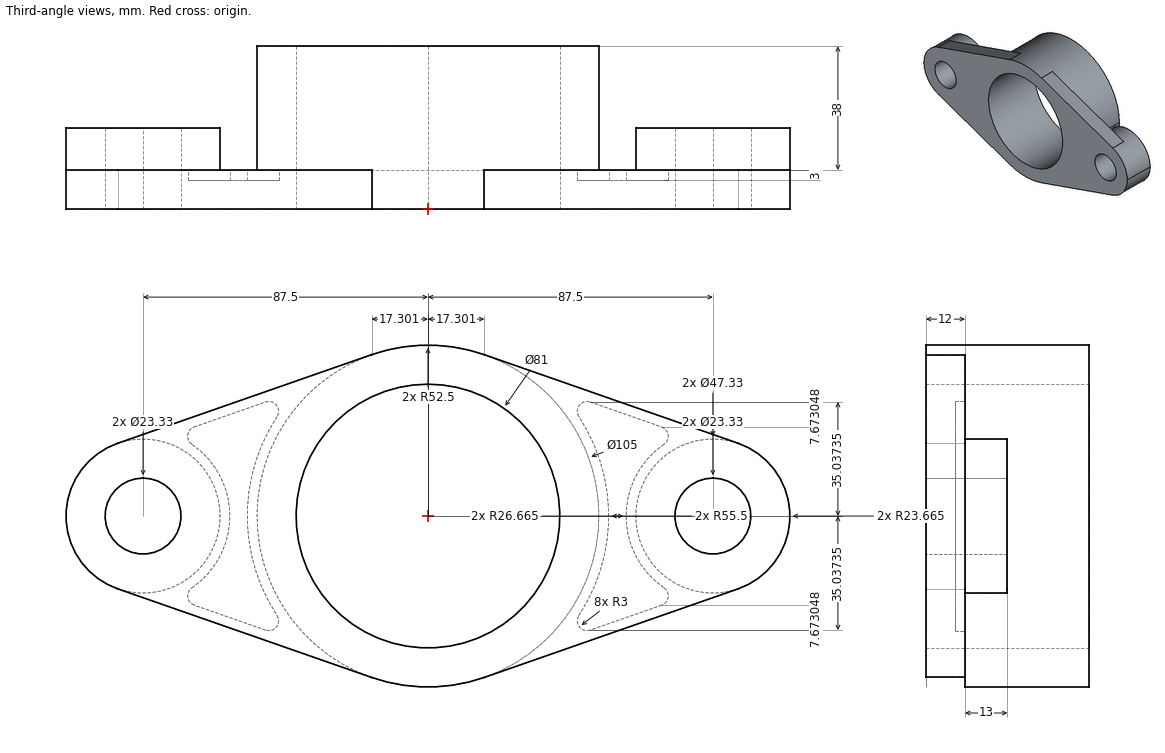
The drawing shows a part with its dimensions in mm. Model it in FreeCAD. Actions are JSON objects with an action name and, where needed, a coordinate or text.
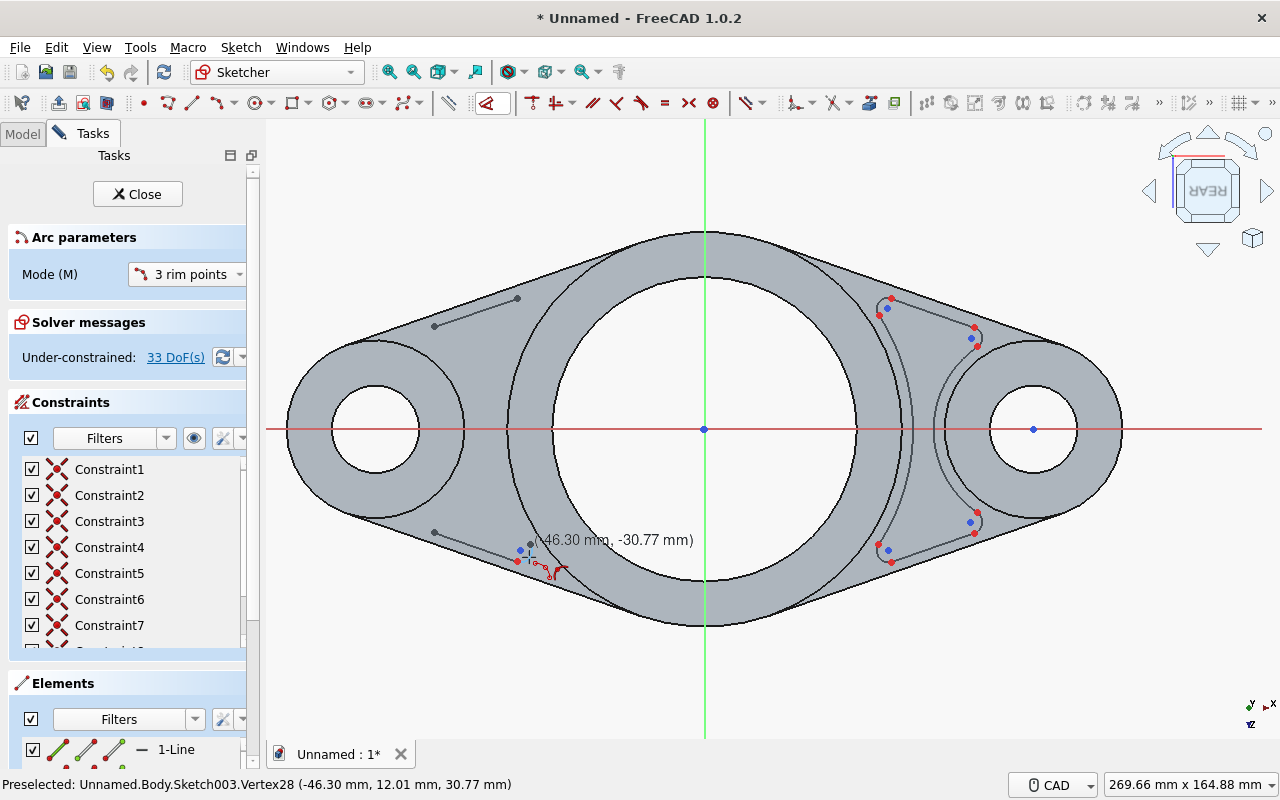
{"action": "left_click", "coordinate": [530, 314]}
{"action": "left_click", "coordinate": [497, 405]}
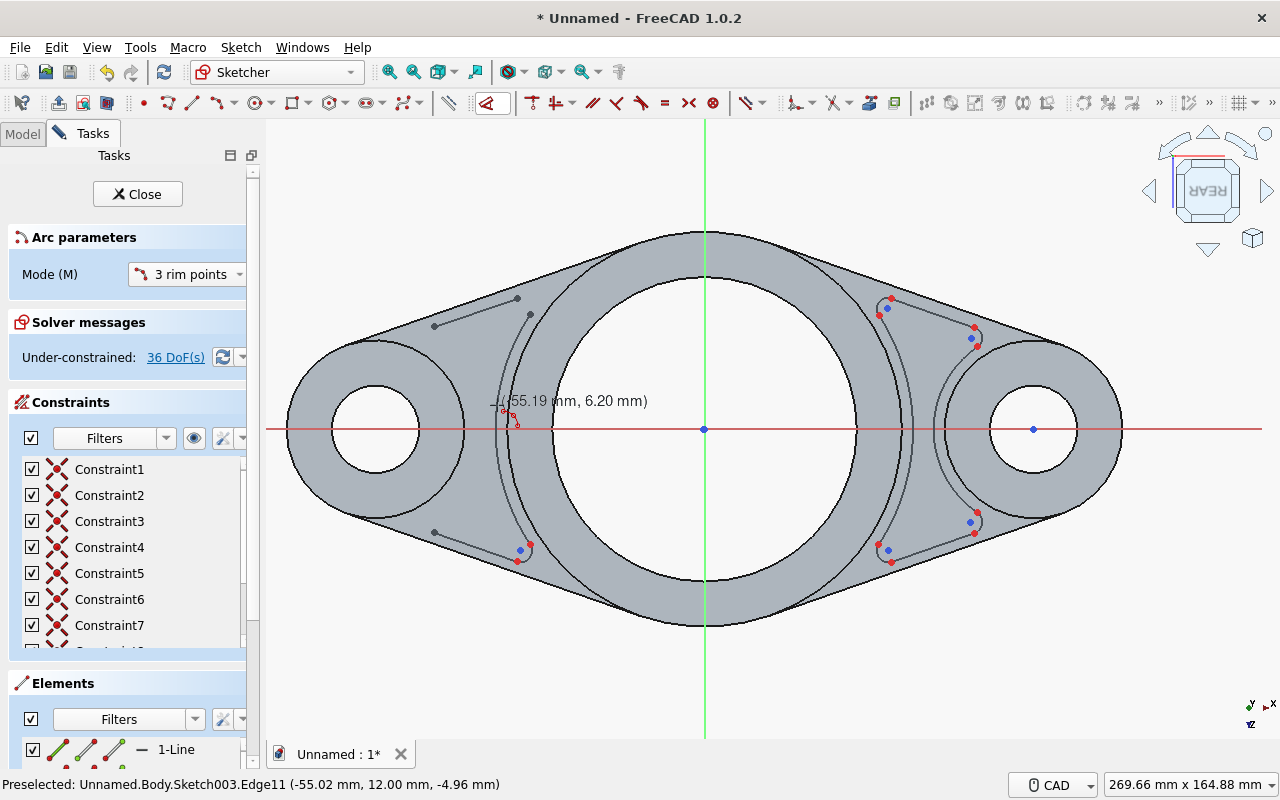
{"action": "left_click", "coordinate": [530, 315]}
{"action": "left_click", "coordinate": [517, 299]}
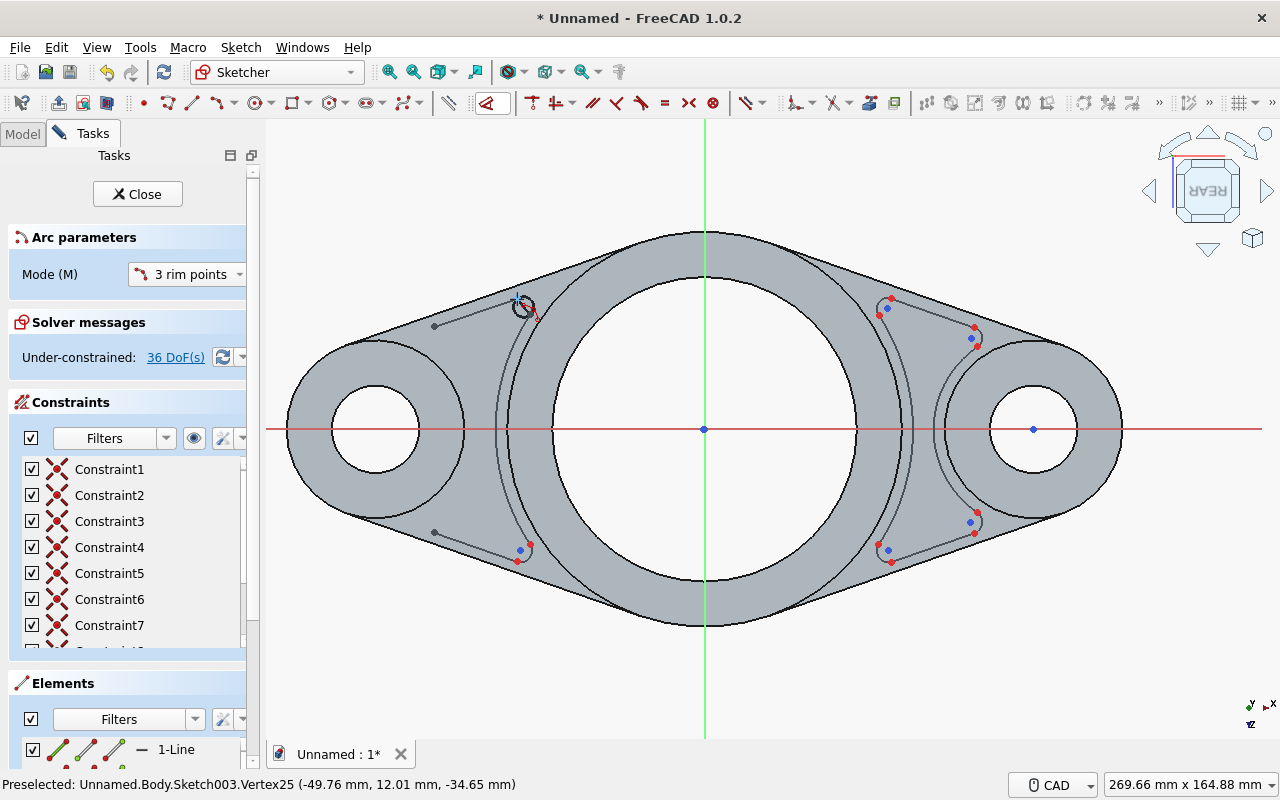
{"action": "scroll", "coordinate": [530, 301], "scroll_direction": "up", "scroll_amount": 4}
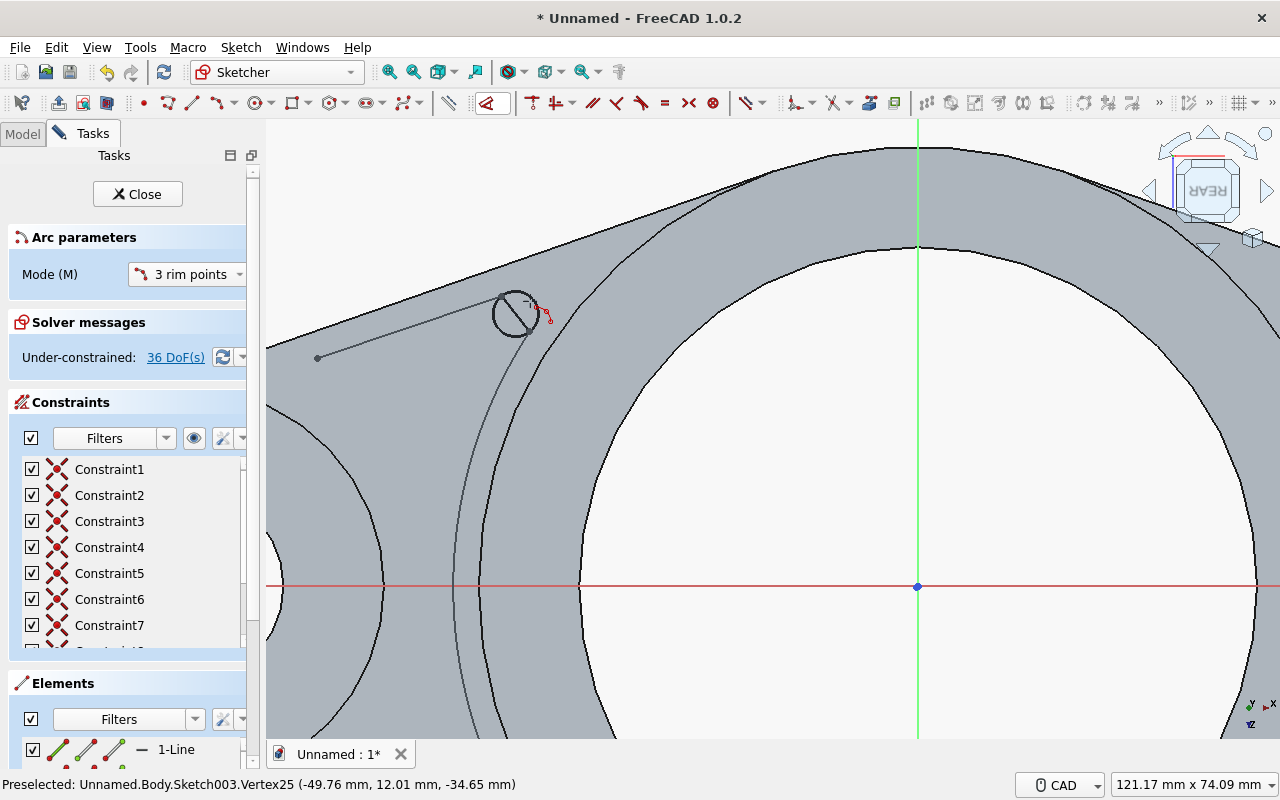
{"action": "left_click", "coordinate": [529, 301]}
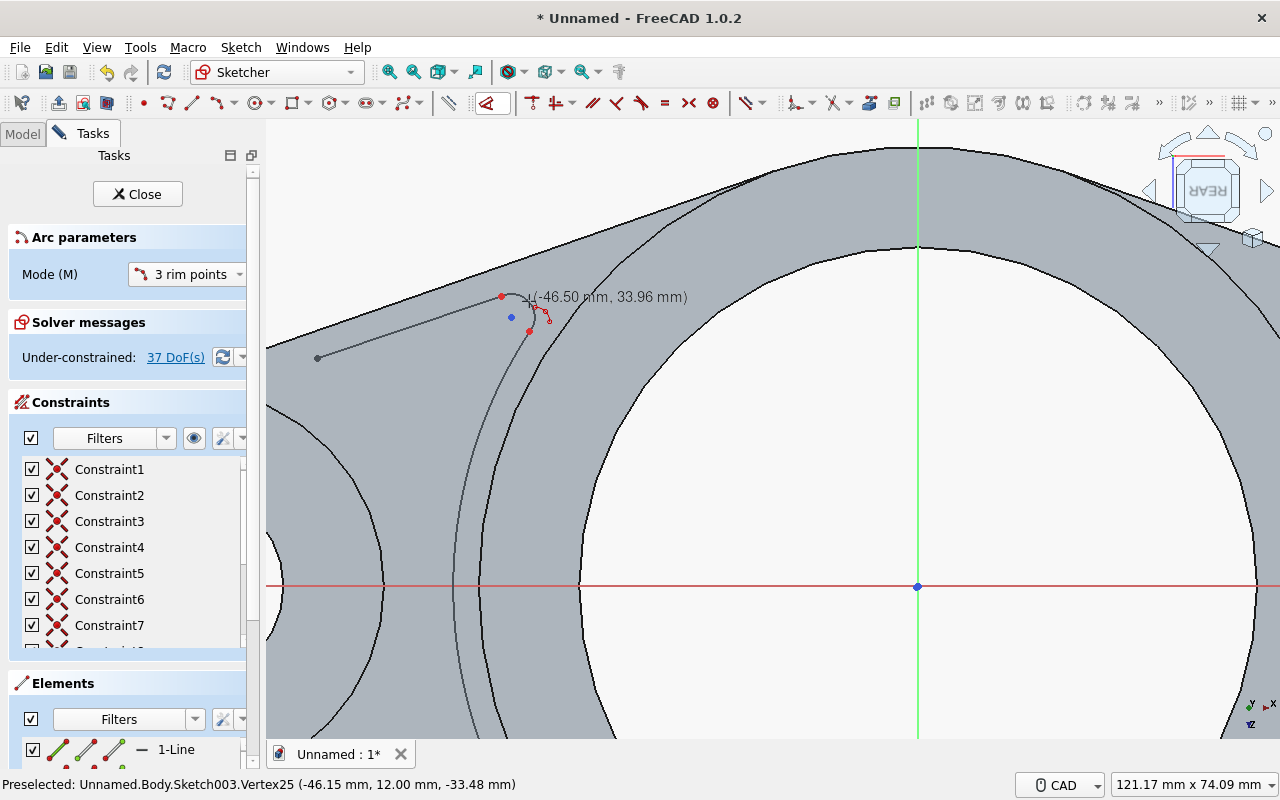
{"action": "left_click", "coordinate": [317, 359]}
{"action": "left_click", "coordinate": [311, 402]}
{"action": "left_click", "coordinate": [301, 378]}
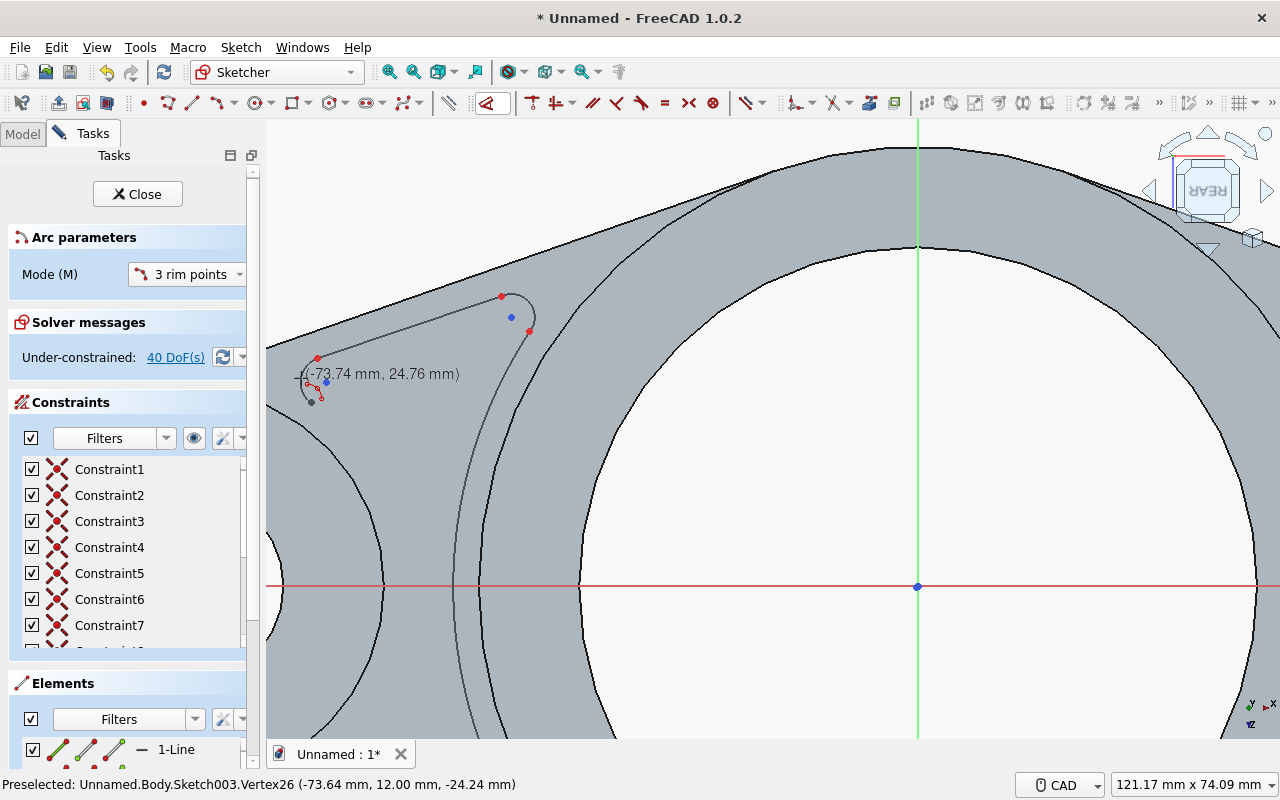
{"action": "left_click", "coordinate": [311, 403]}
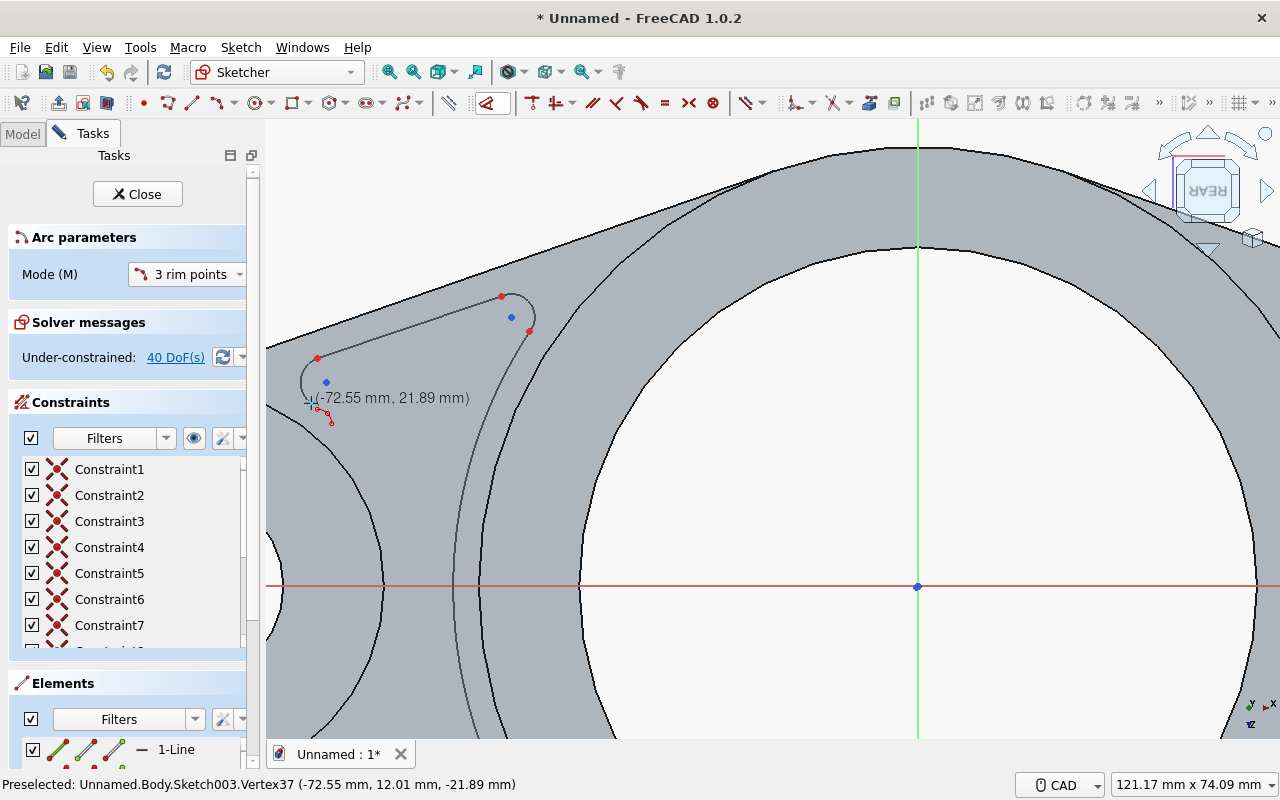
{"action": "scroll", "coordinate": [530, 301], "scroll_direction": "down", "scroll_amount": 4}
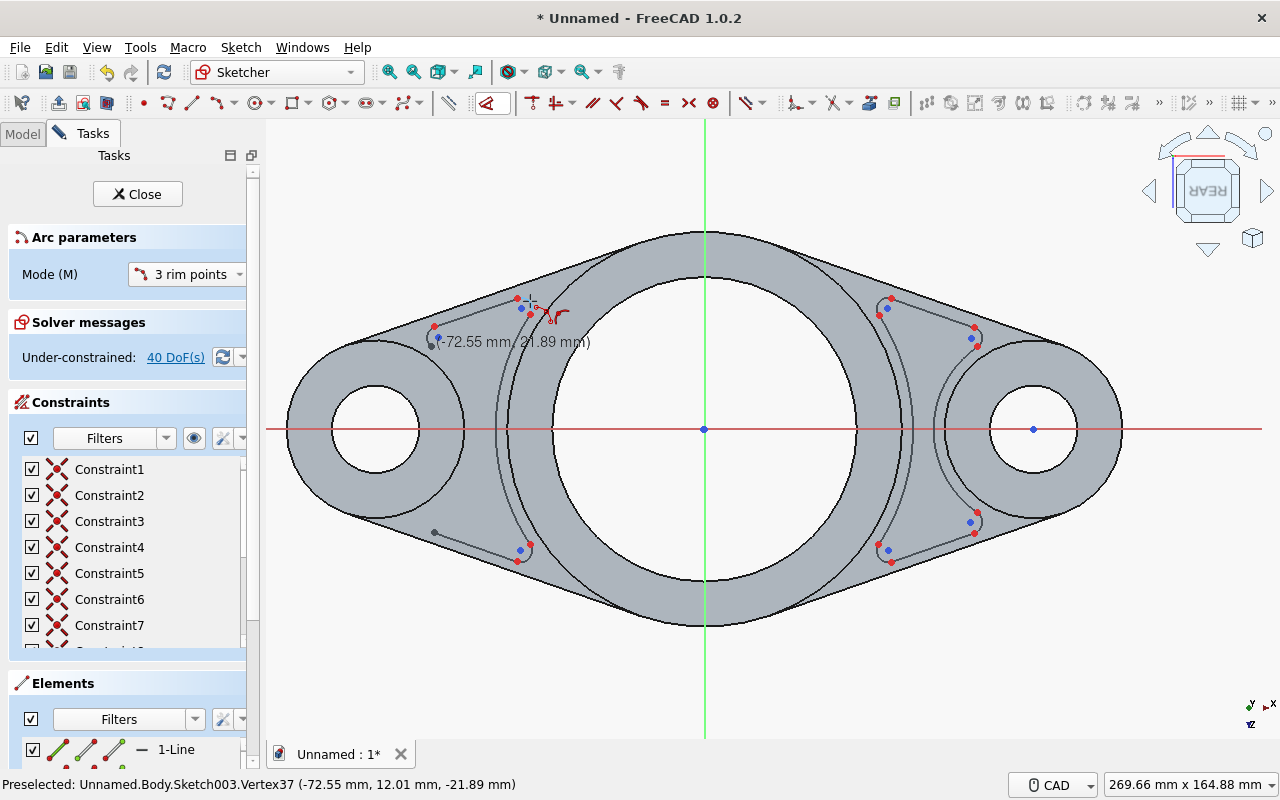
{"action": "left_click", "coordinate": [432, 512]}
{"action": "left_click", "coordinate": [474, 449]}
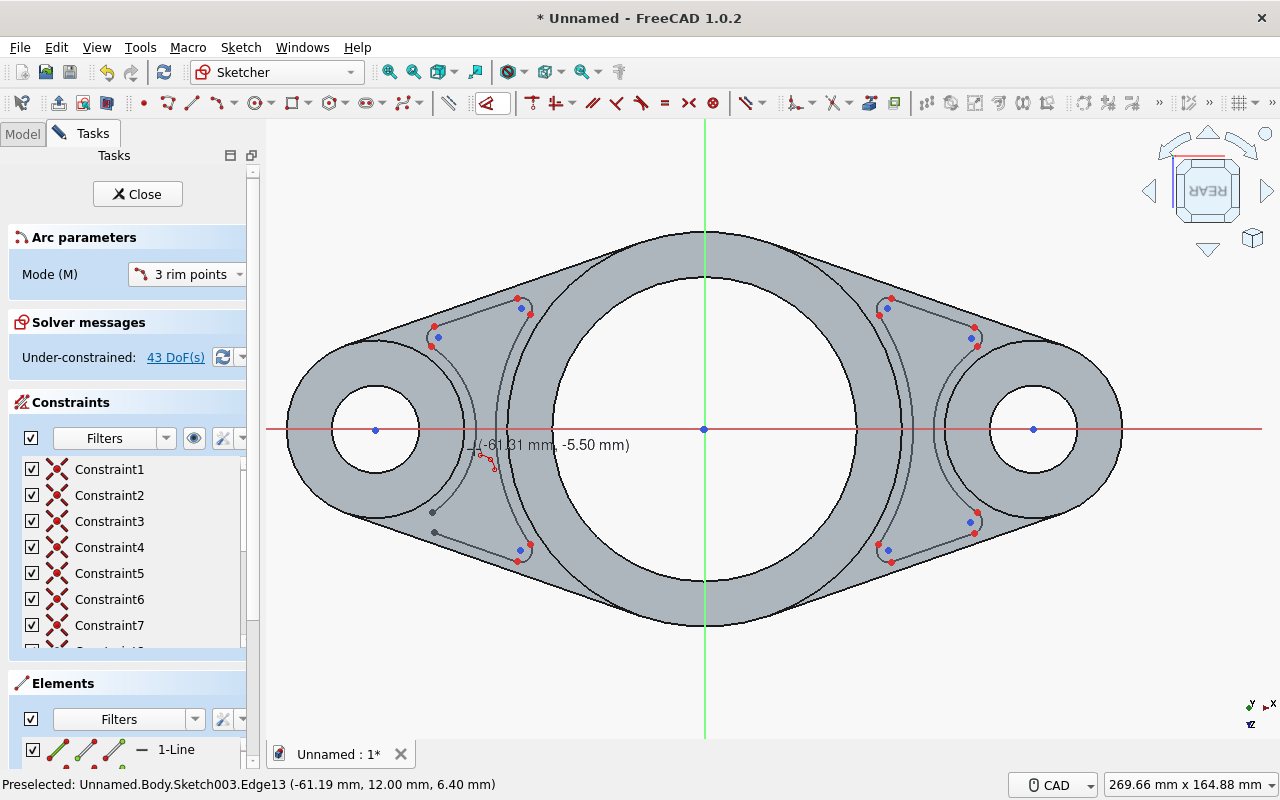
{"action": "left_click", "coordinate": [432, 513]}
{"action": "left_click", "coordinate": [434, 533]}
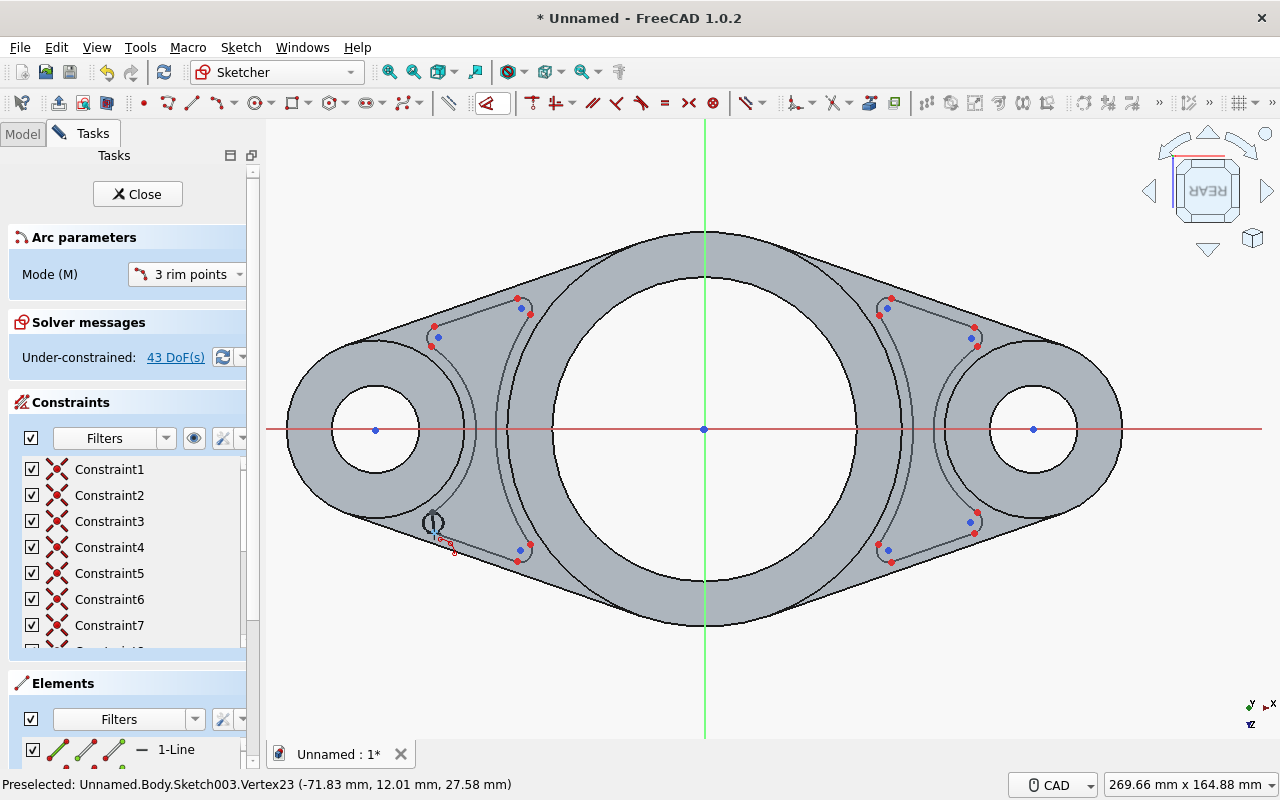
{"action": "scroll", "coordinate": [427, 523], "scroll_direction": "up", "scroll_amount": 5}